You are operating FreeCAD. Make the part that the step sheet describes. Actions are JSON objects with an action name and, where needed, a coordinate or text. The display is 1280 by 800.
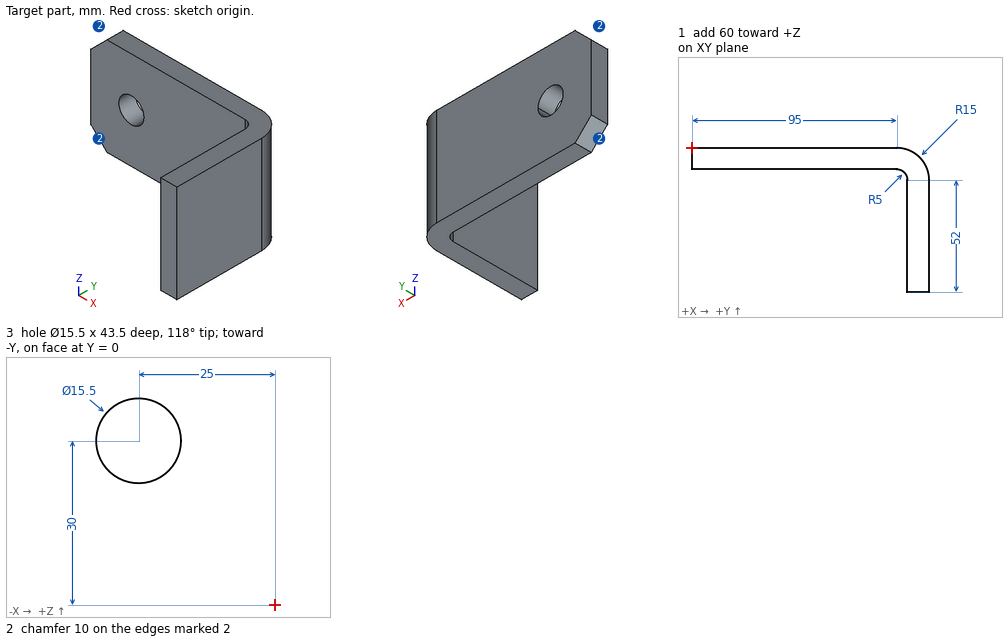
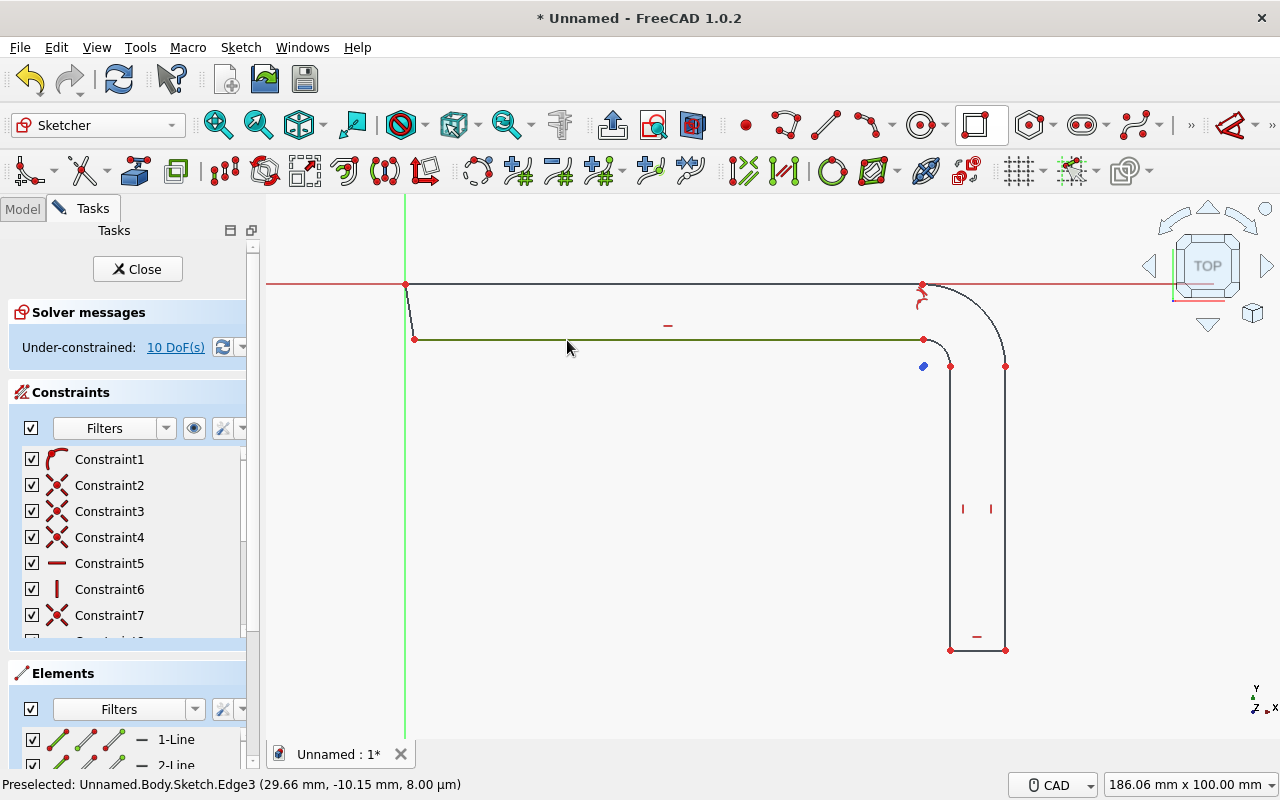
{"action": "left_click", "coordinate": [947, 354]}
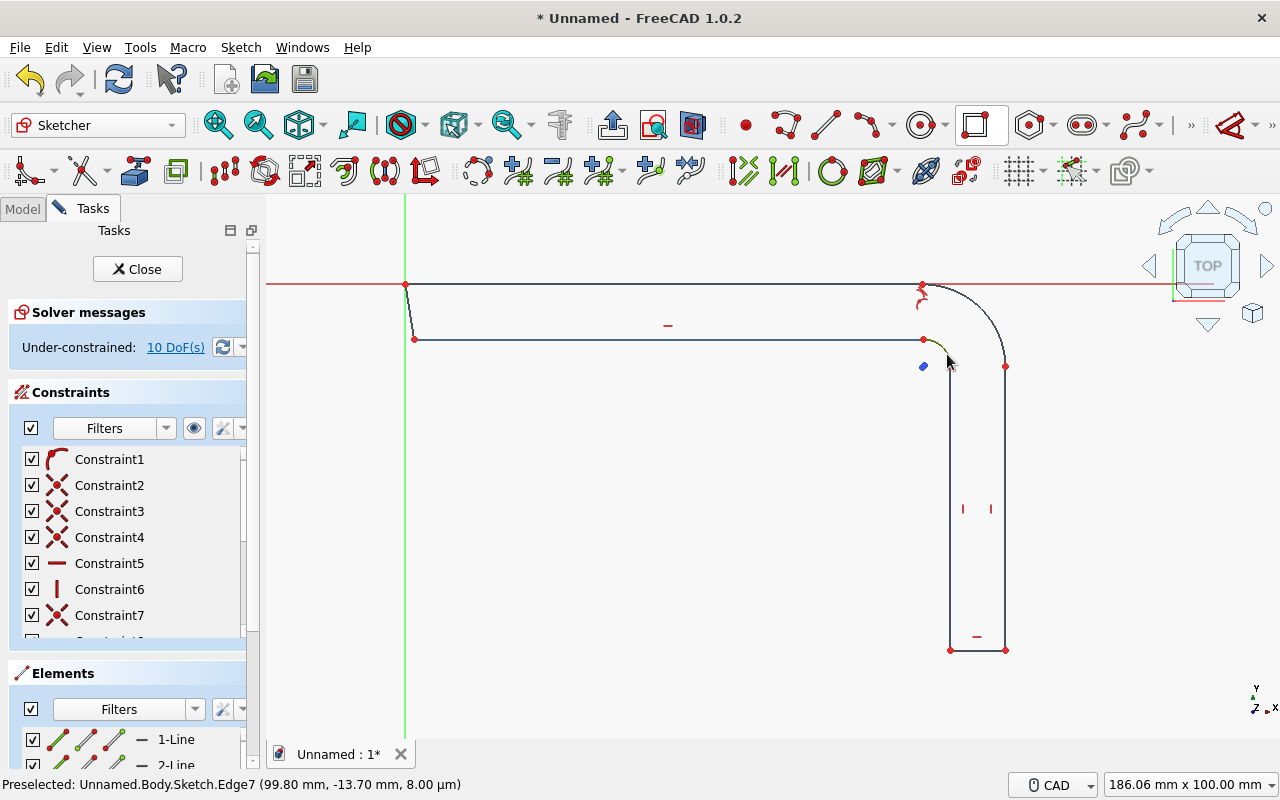
{"action": "key", "text": "t"}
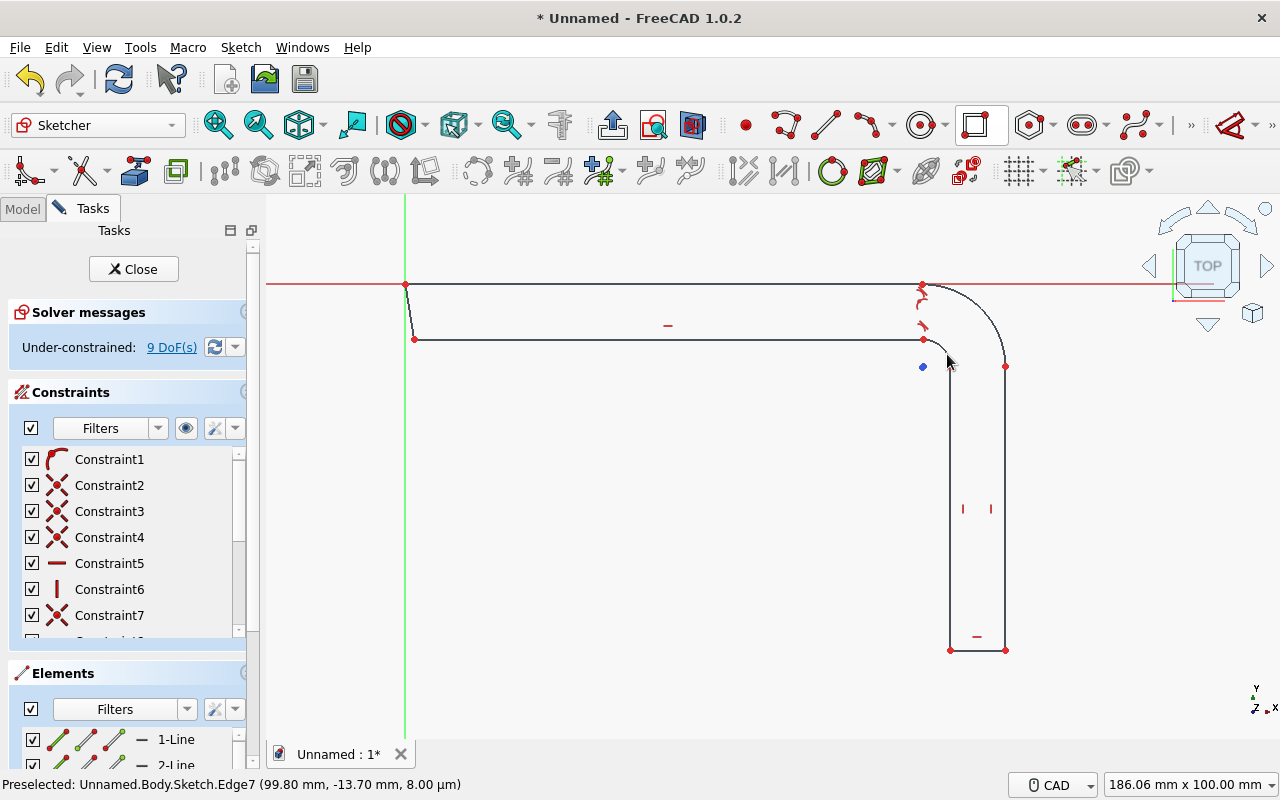
{"action": "left_click", "coordinate": [950, 452]}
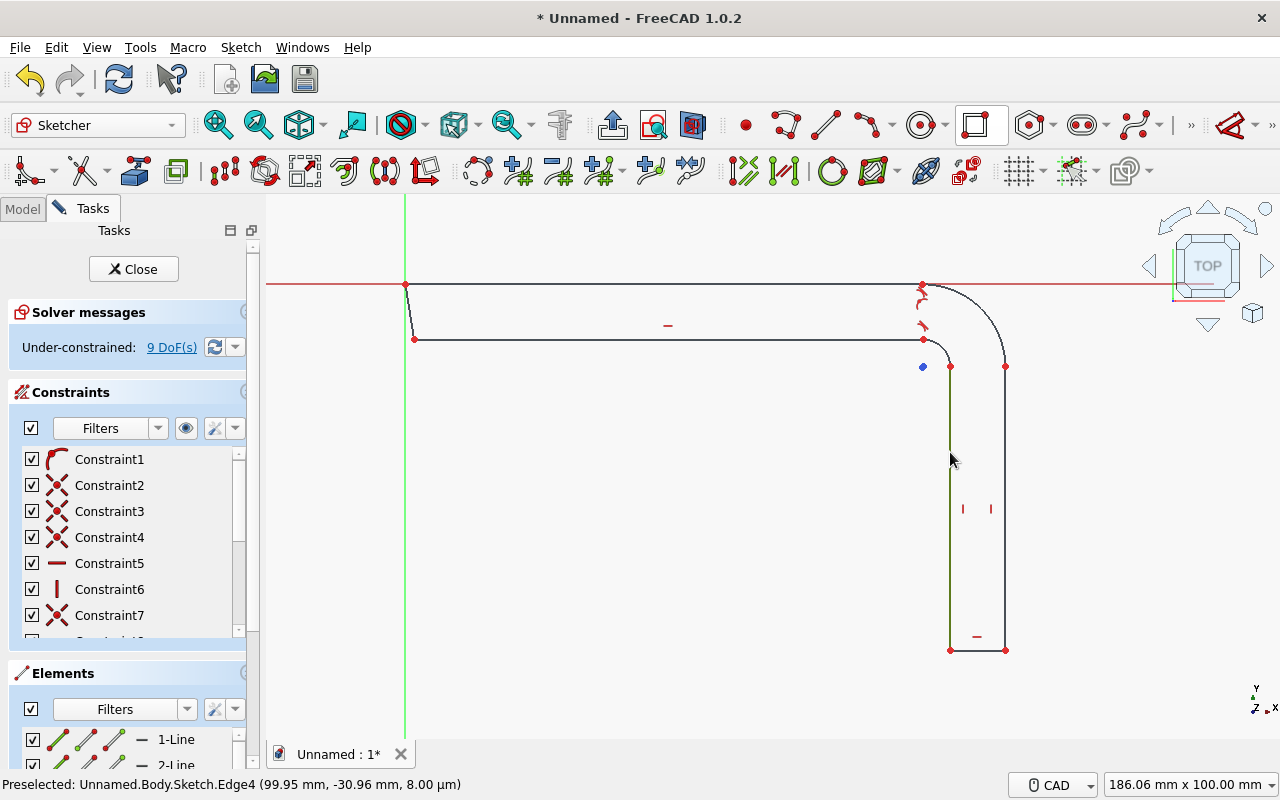
{"action": "left_click", "coordinate": [947, 354]}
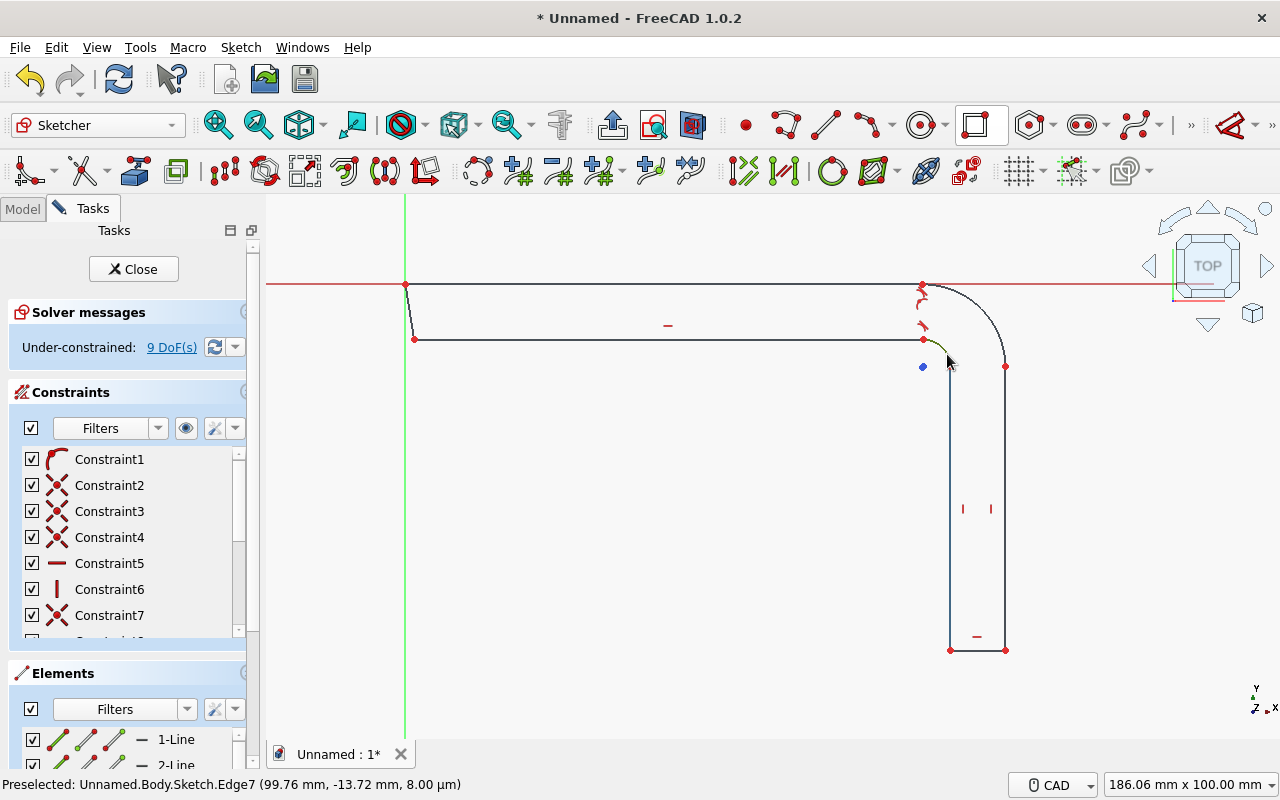
{"action": "key", "text": "t"}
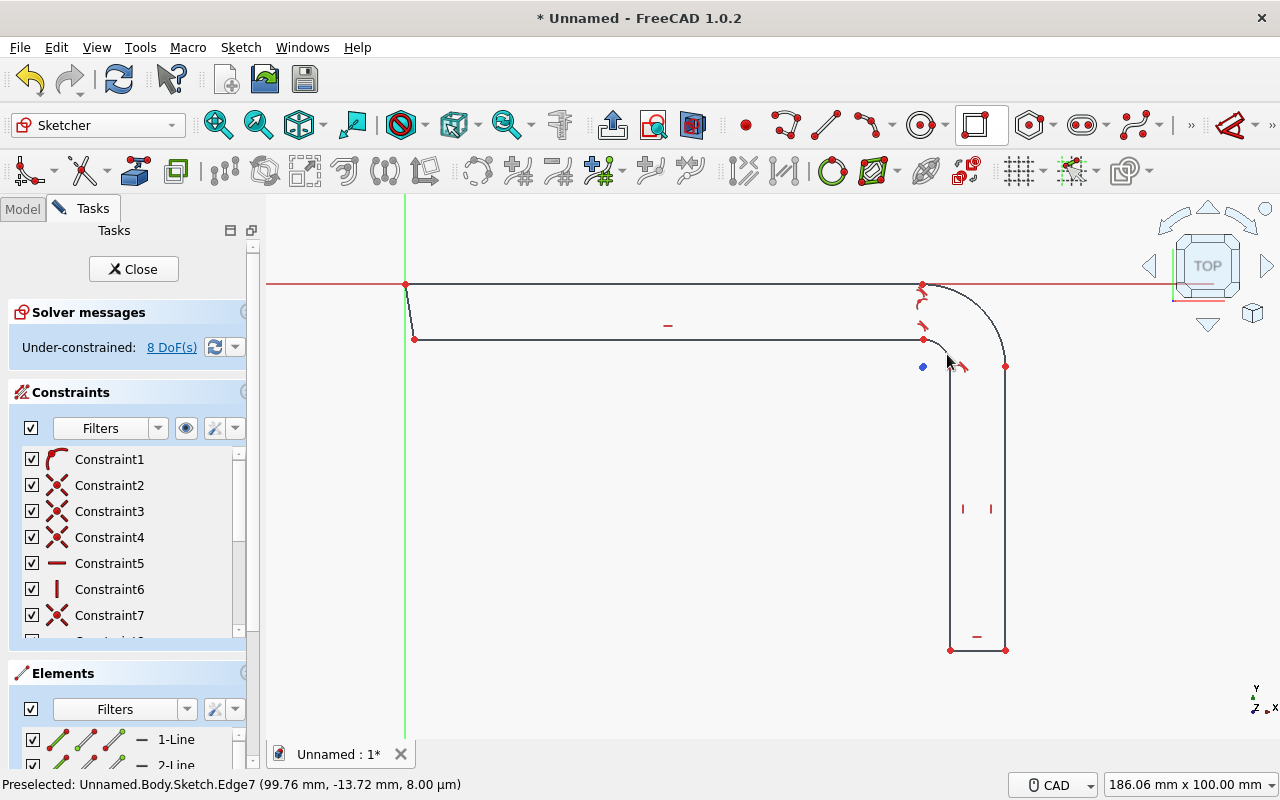
{"action": "left_click", "coordinate": [1005, 565]}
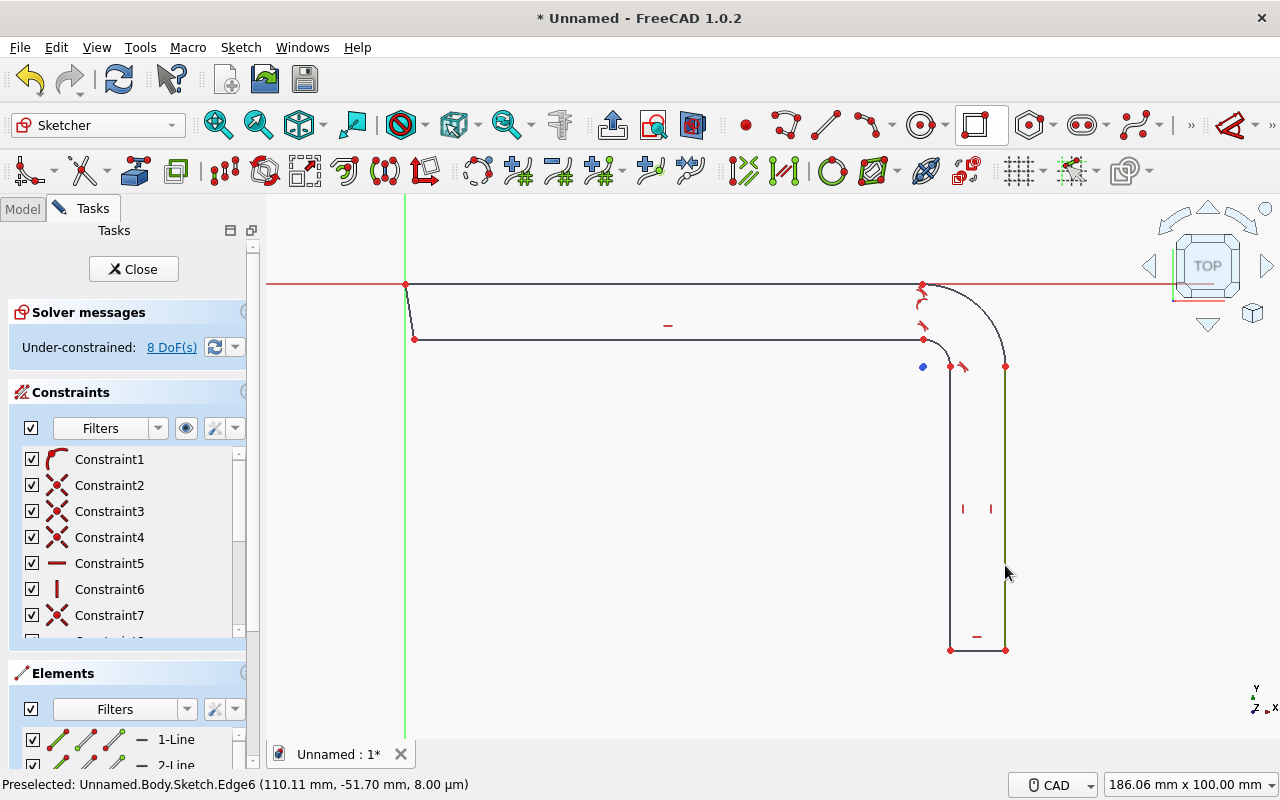
{"action": "left_click", "coordinate": [996, 329]}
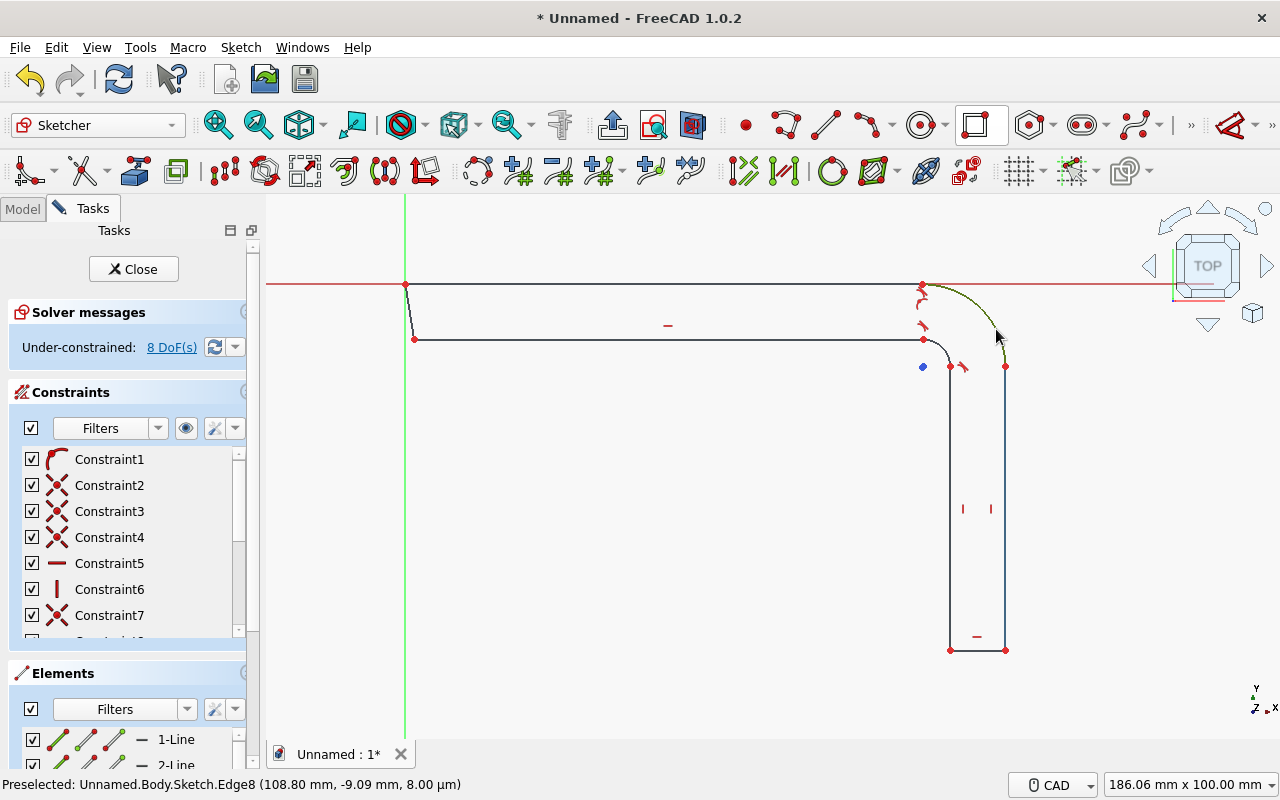
{"action": "key", "text": "t"}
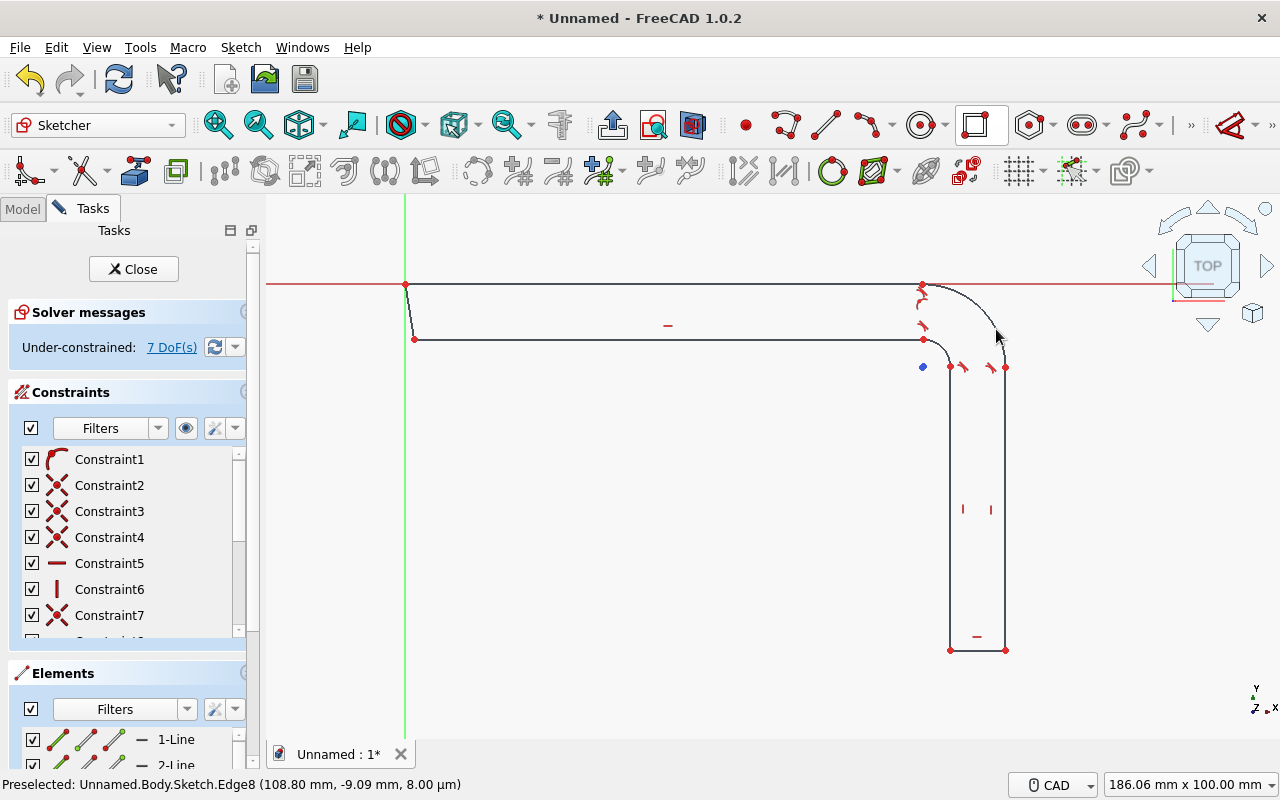
{"action": "left_click", "coordinate": [408, 301]}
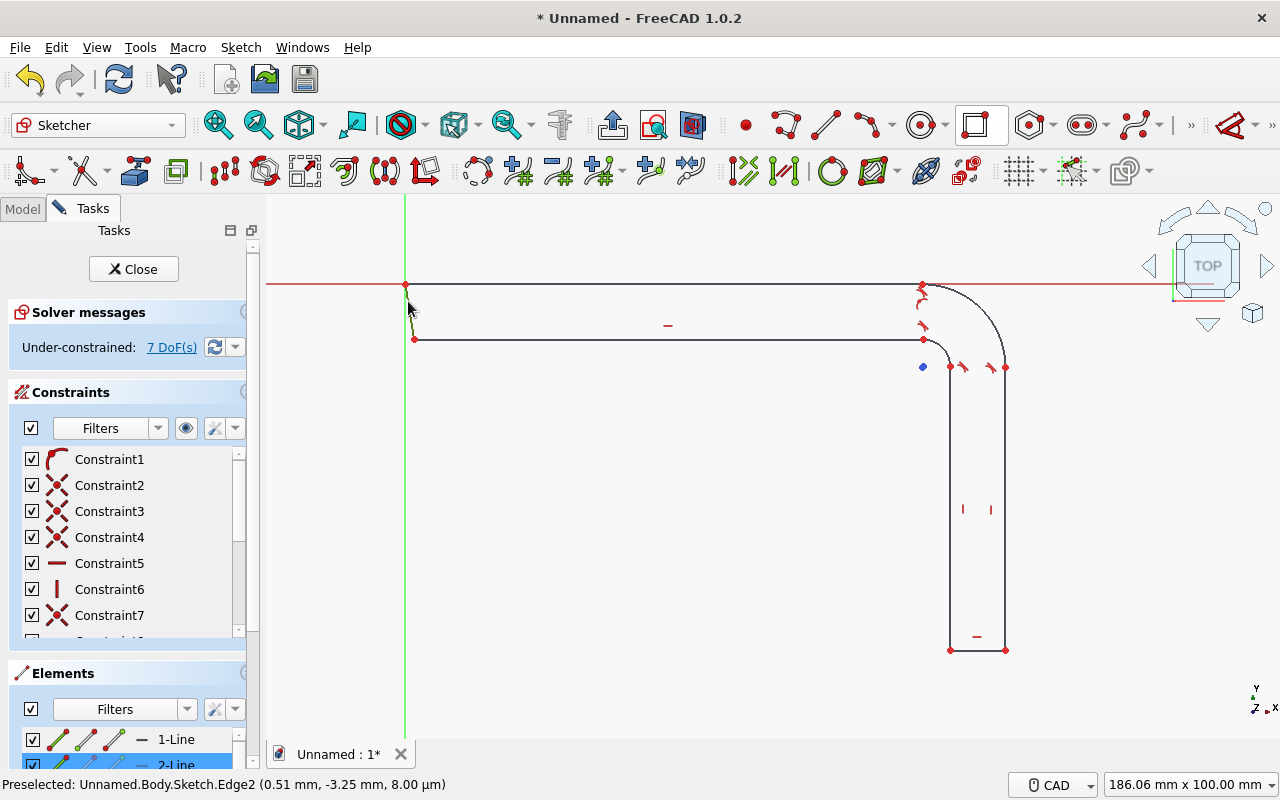
{"action": "key", "text": "v"}